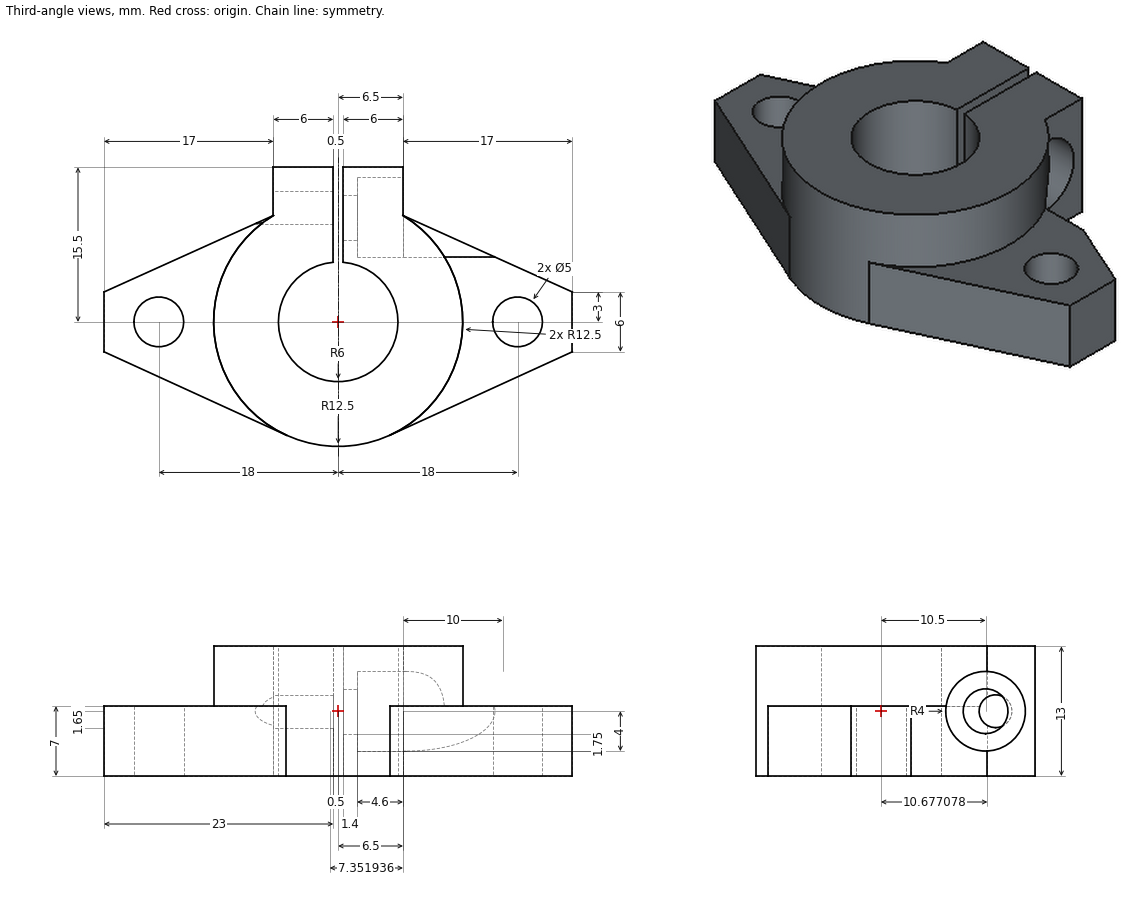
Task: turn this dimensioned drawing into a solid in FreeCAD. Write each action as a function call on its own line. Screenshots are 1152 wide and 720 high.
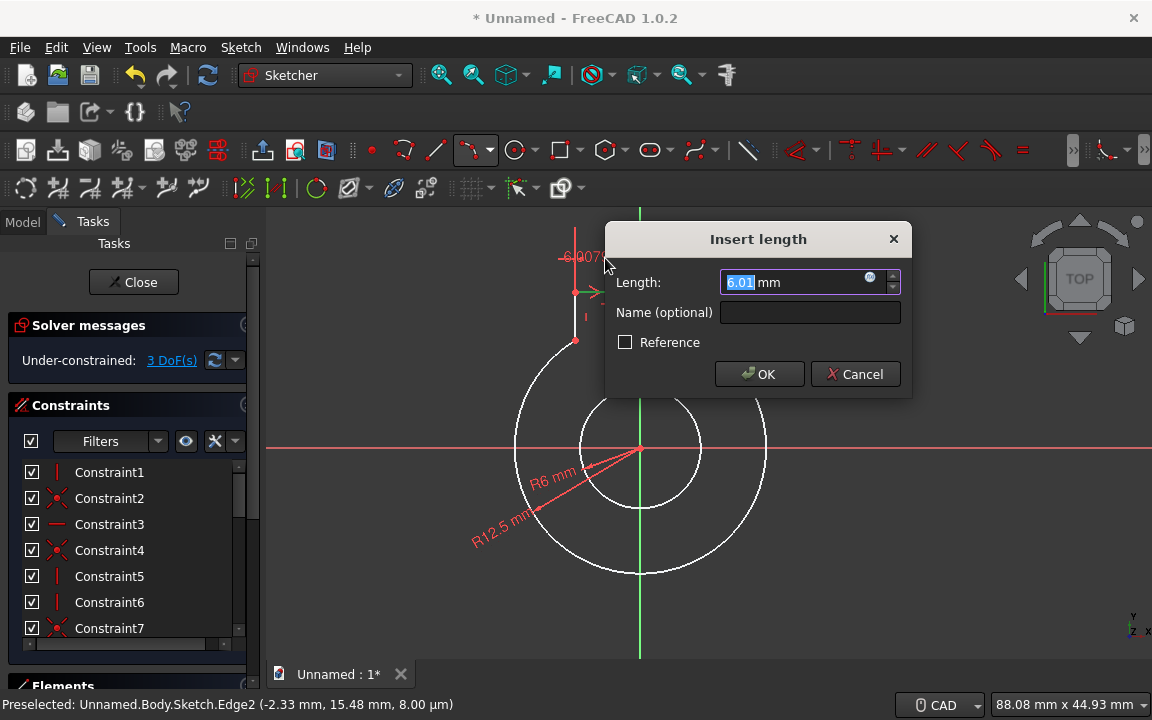
text(6)
key(Return)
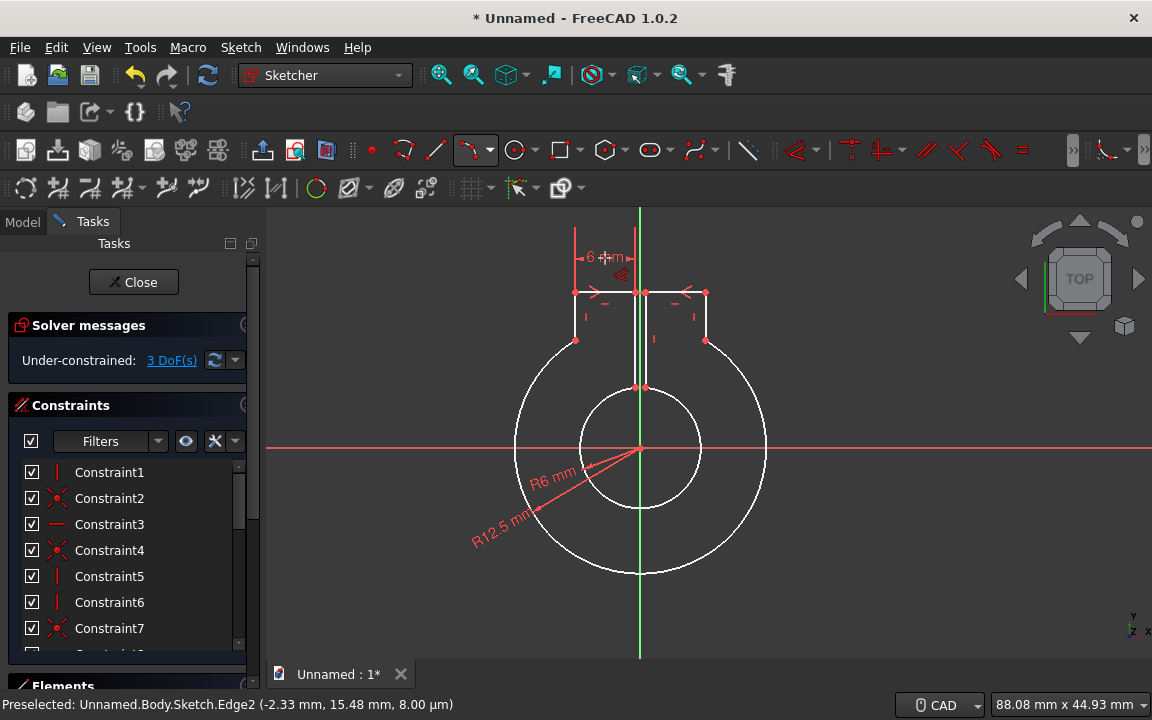
click(688, 292)
click(676, 258)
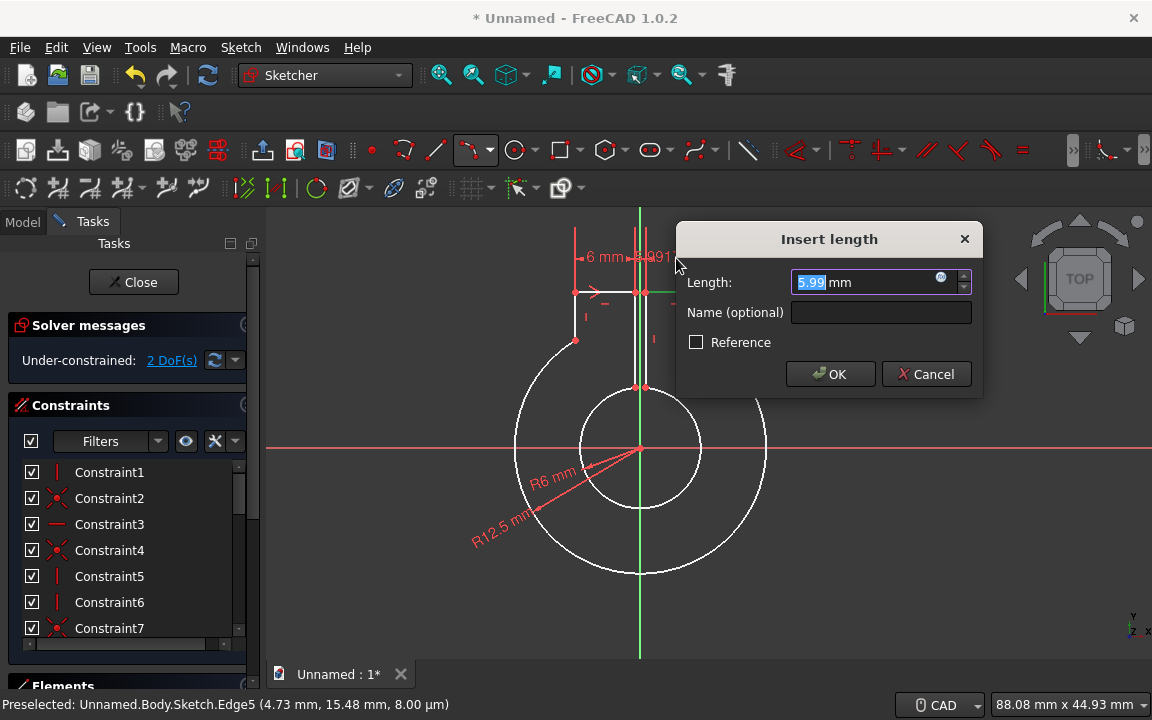
text(6)
key(Return)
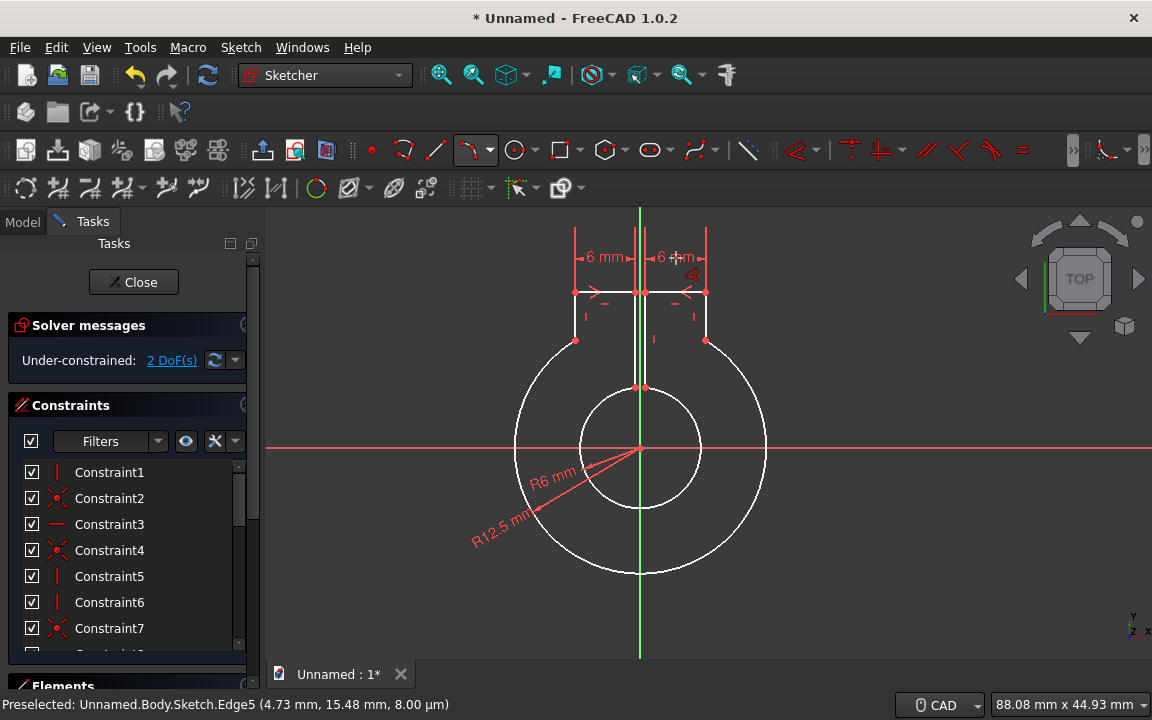
scroll(635, 388, up, 11)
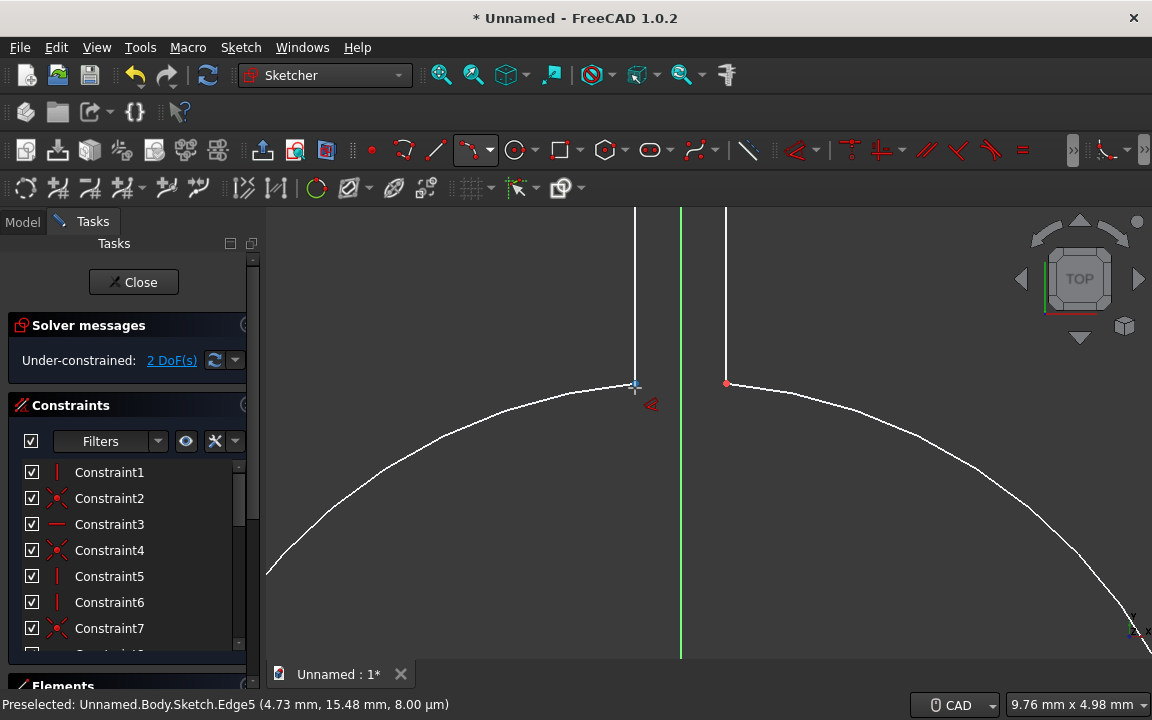
click(635, 384)
click(658, 350)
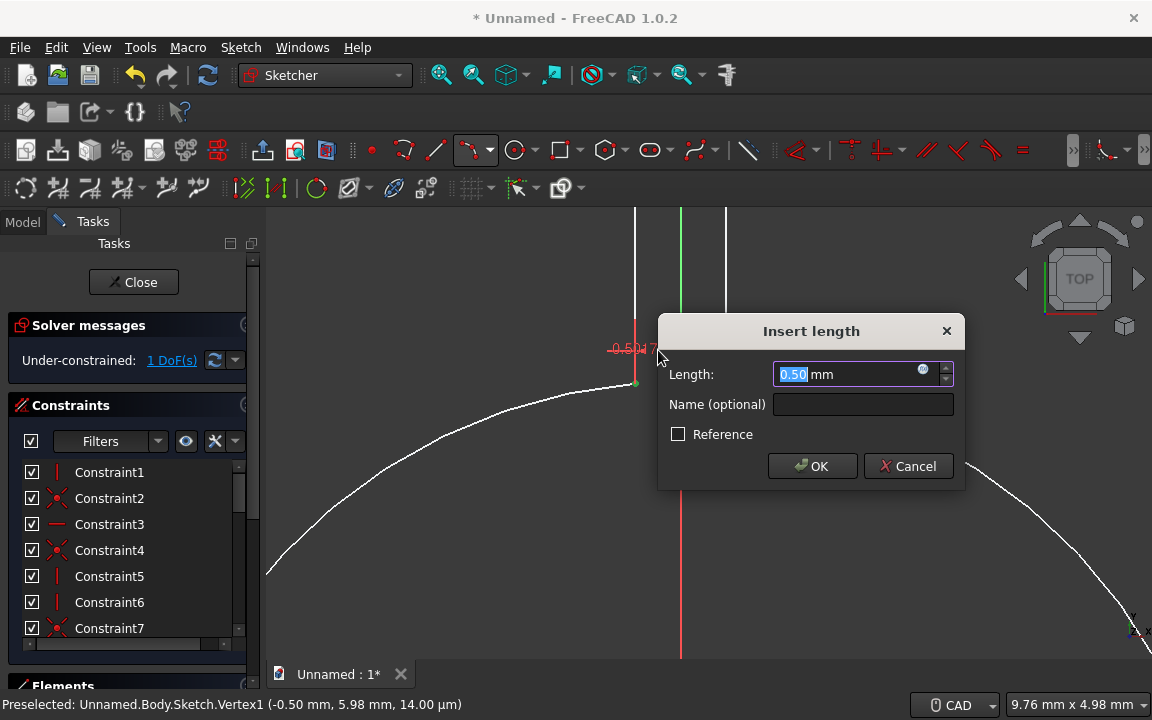
text(0.5)
key(Return)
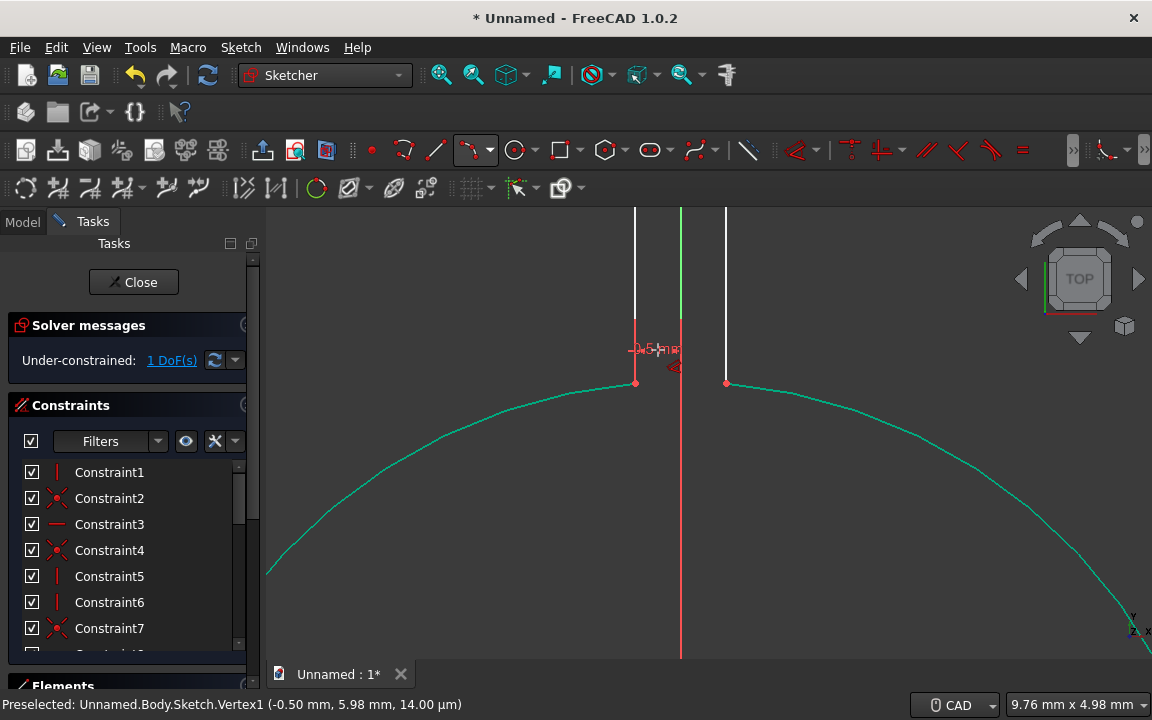
scroll(635, 388, down, 11)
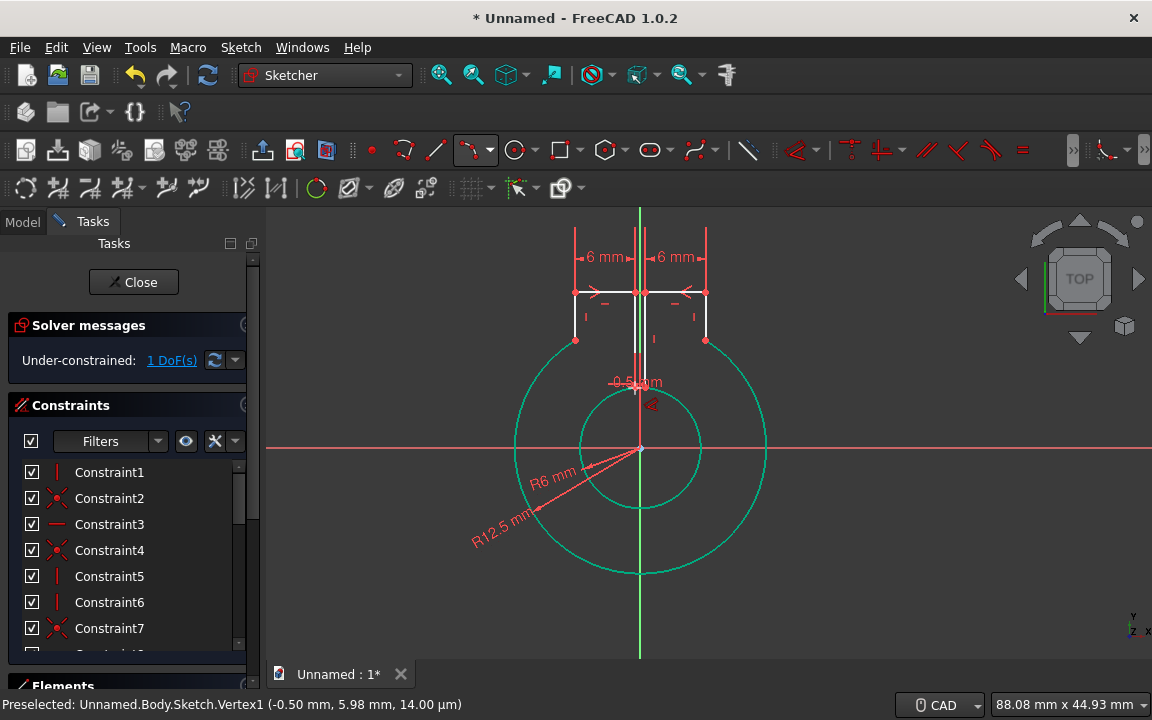
click(635, 292)
click(601, 334)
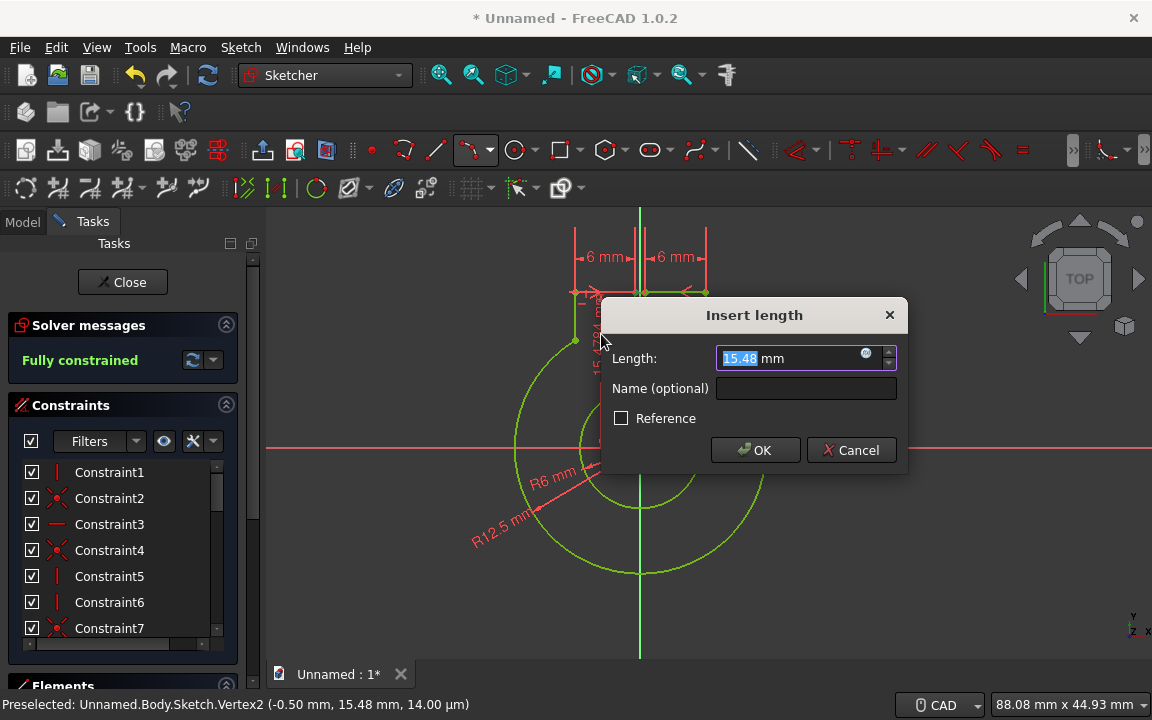
text(15.5)
key(Return)
key(Escape)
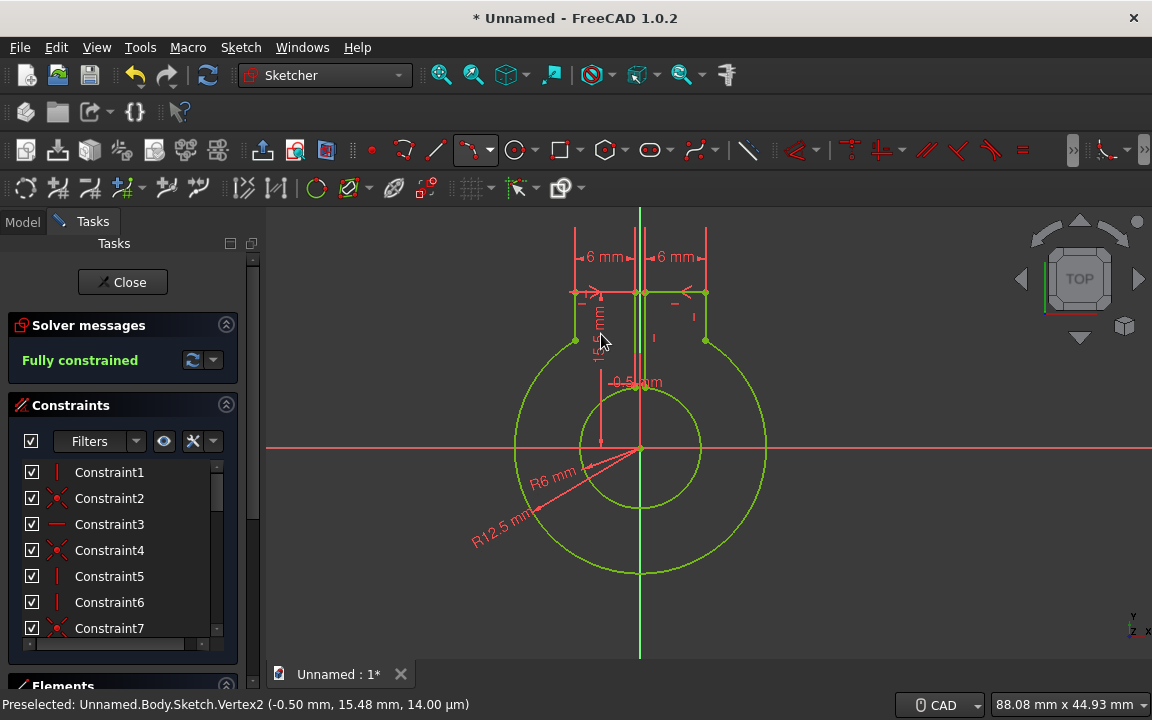
click(123, 282)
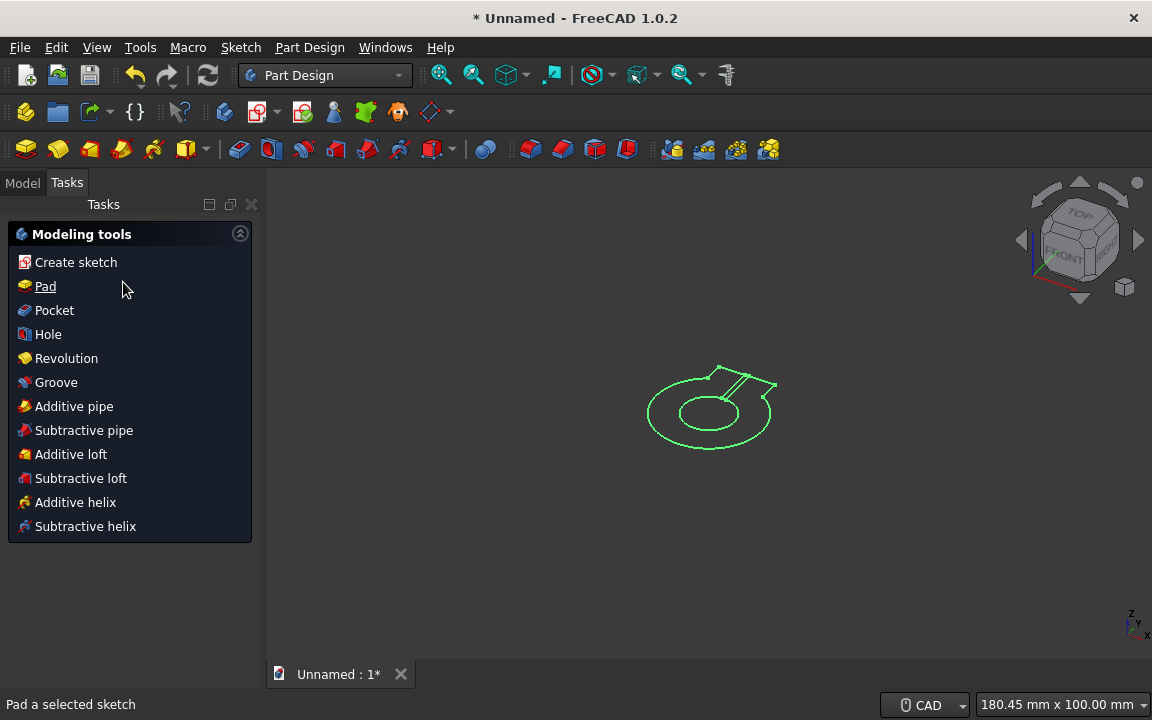
click(26, 150)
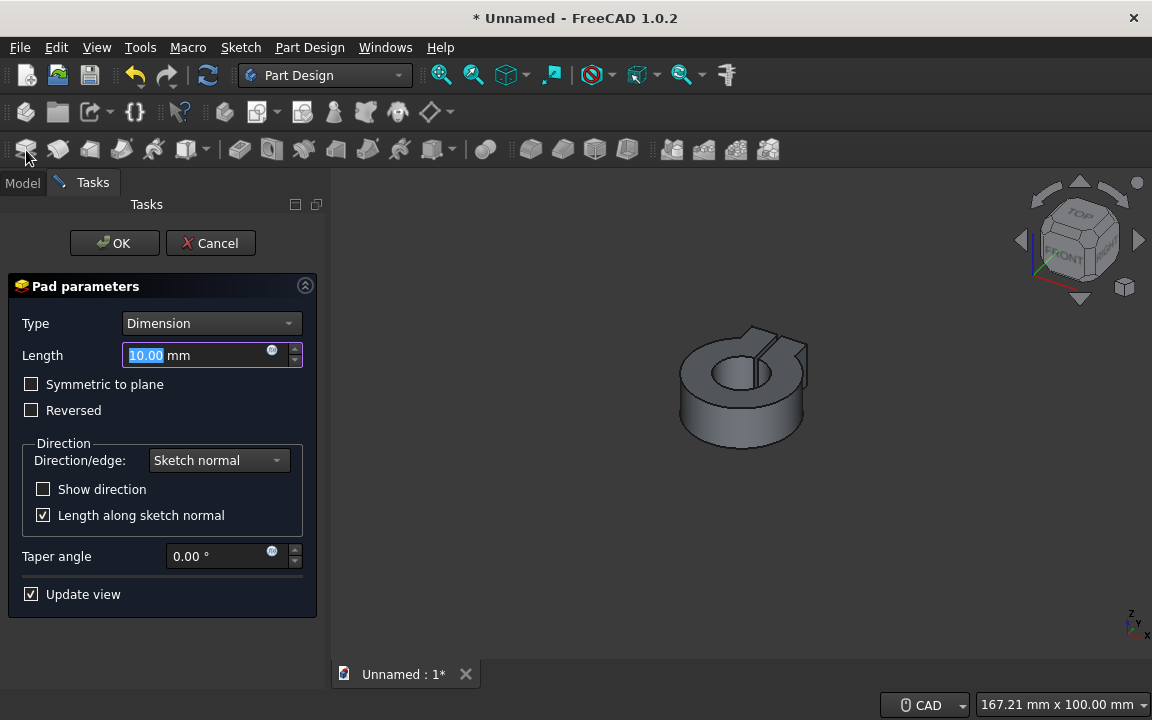
text(13)
key(Tab)